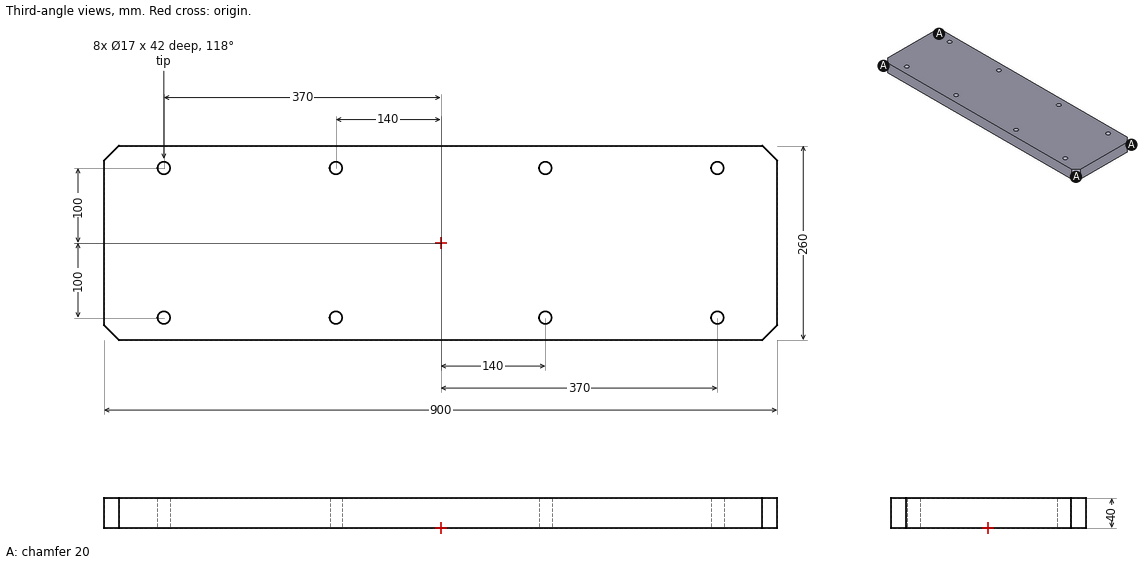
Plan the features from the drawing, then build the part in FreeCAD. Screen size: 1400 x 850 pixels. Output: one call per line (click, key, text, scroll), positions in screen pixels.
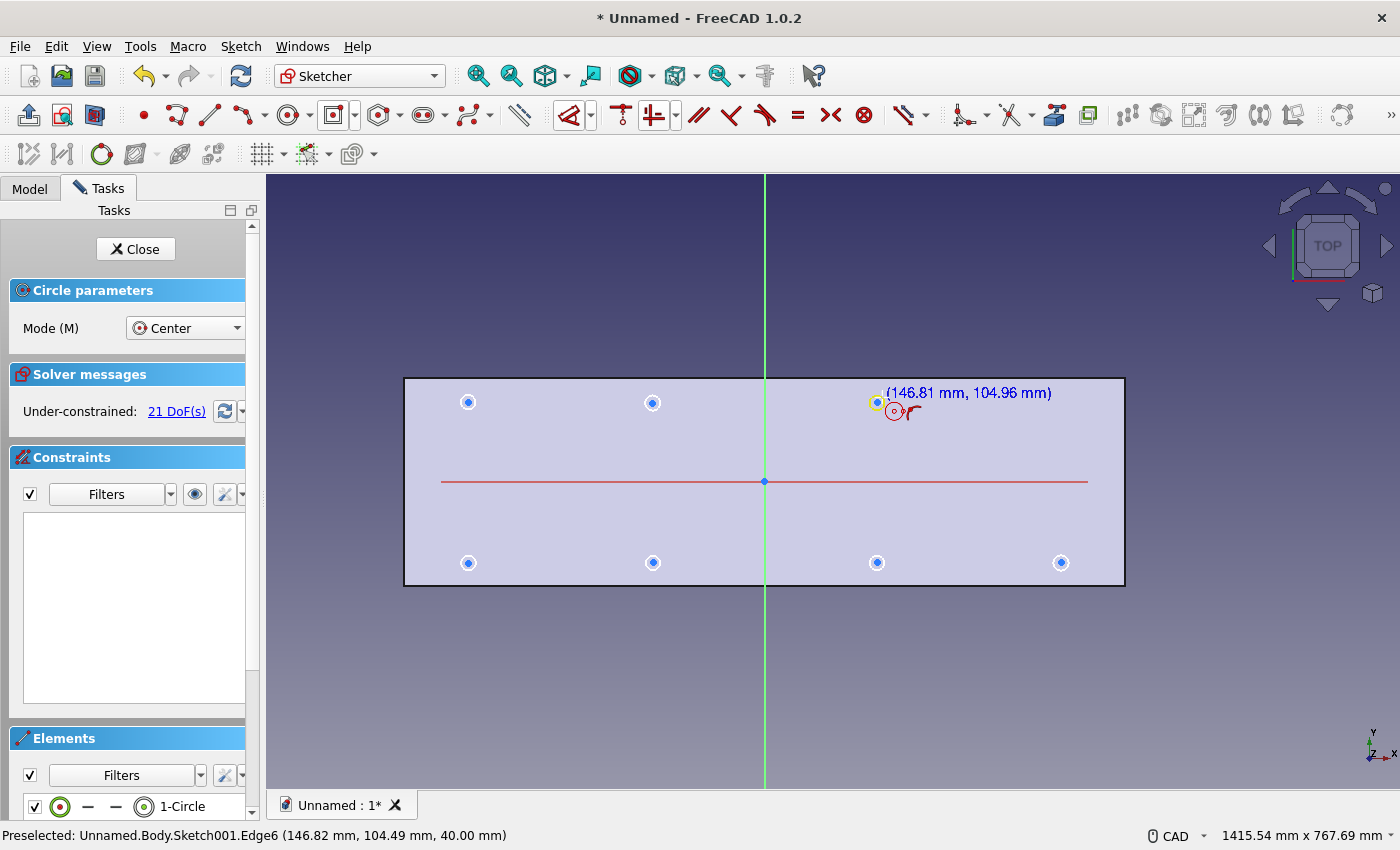
scroll(1061, 402, up, 7)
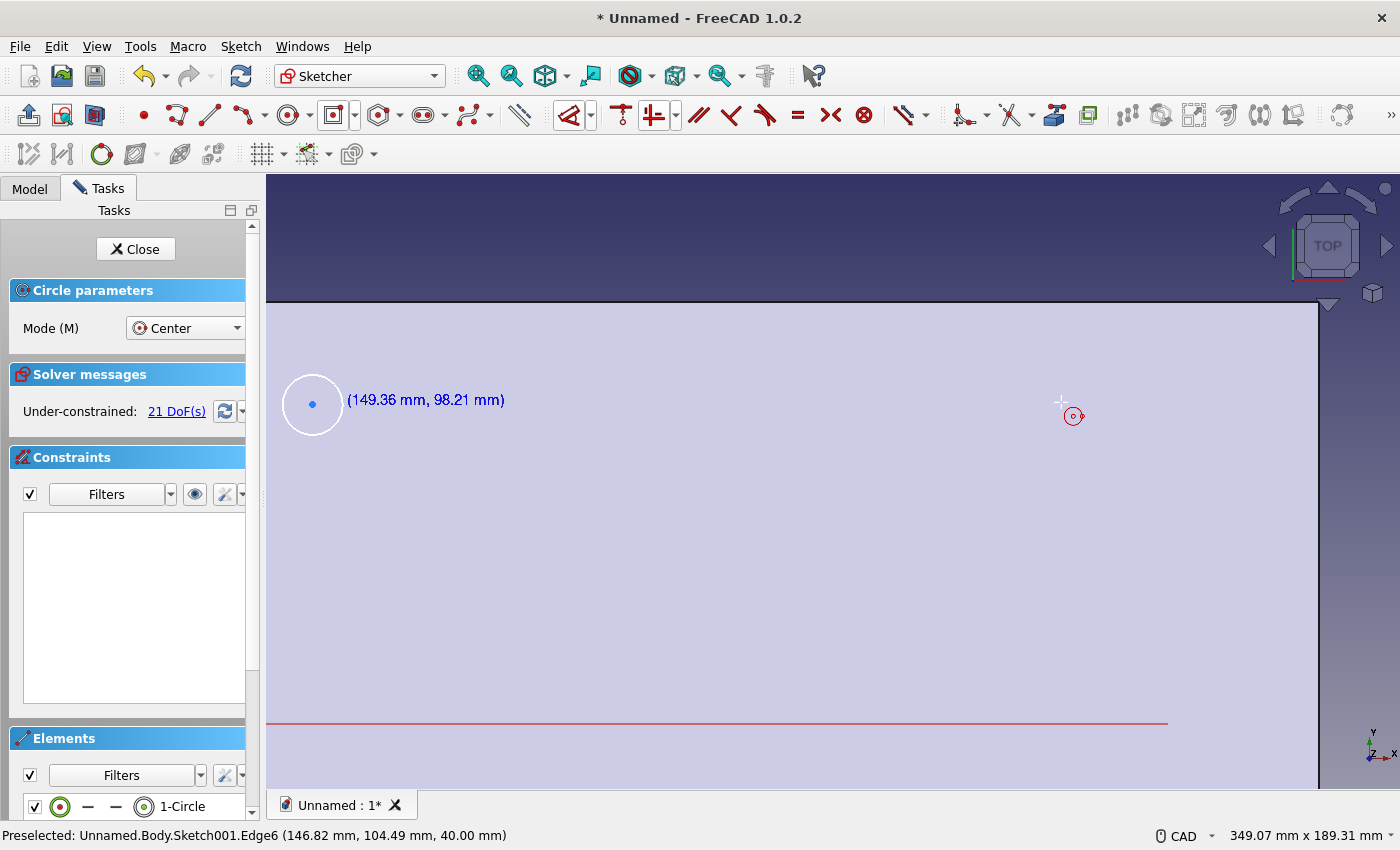
scroll(1061, 402, down, 7)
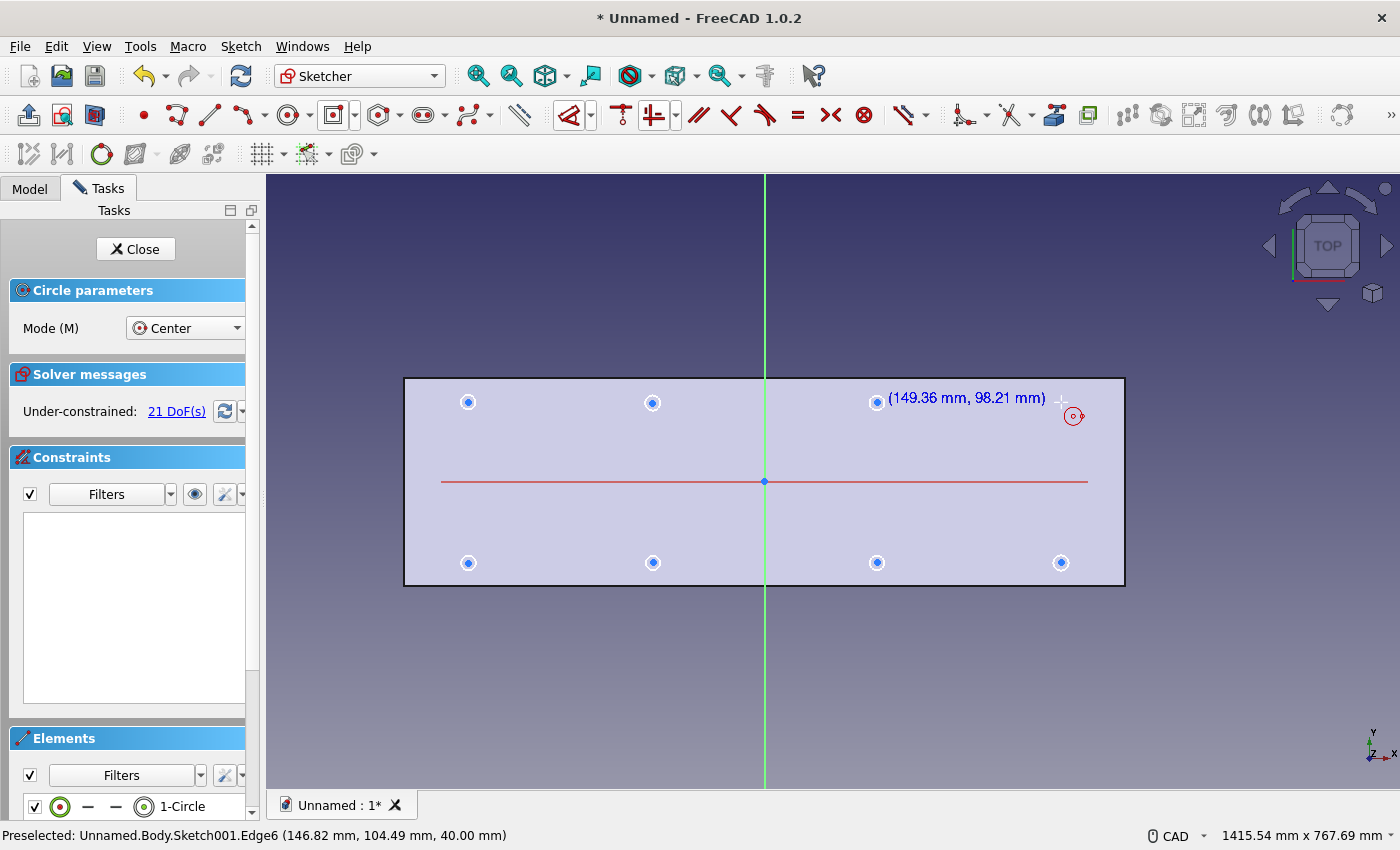
click(1061, 402)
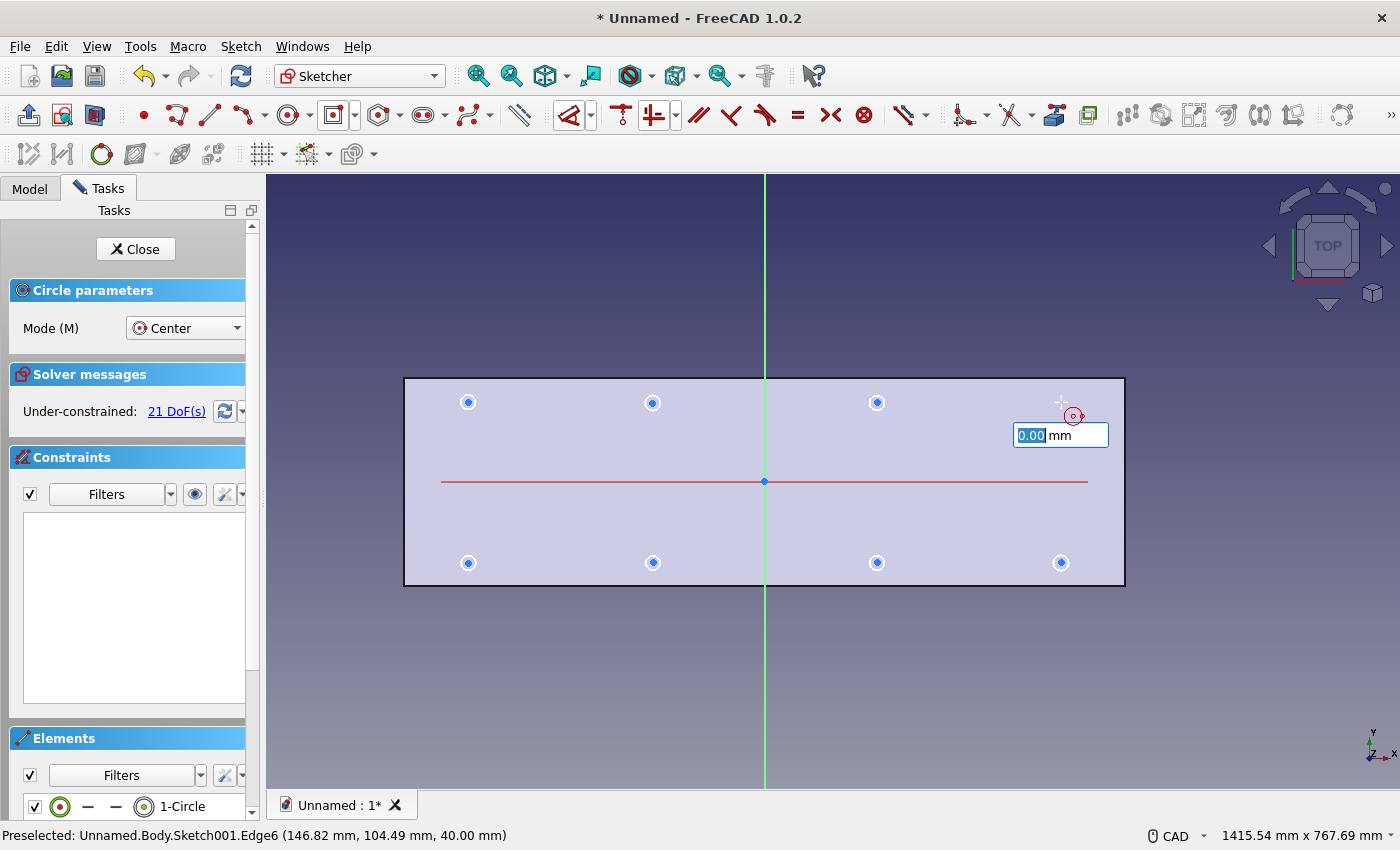
scroll(1066, 397, up, 5)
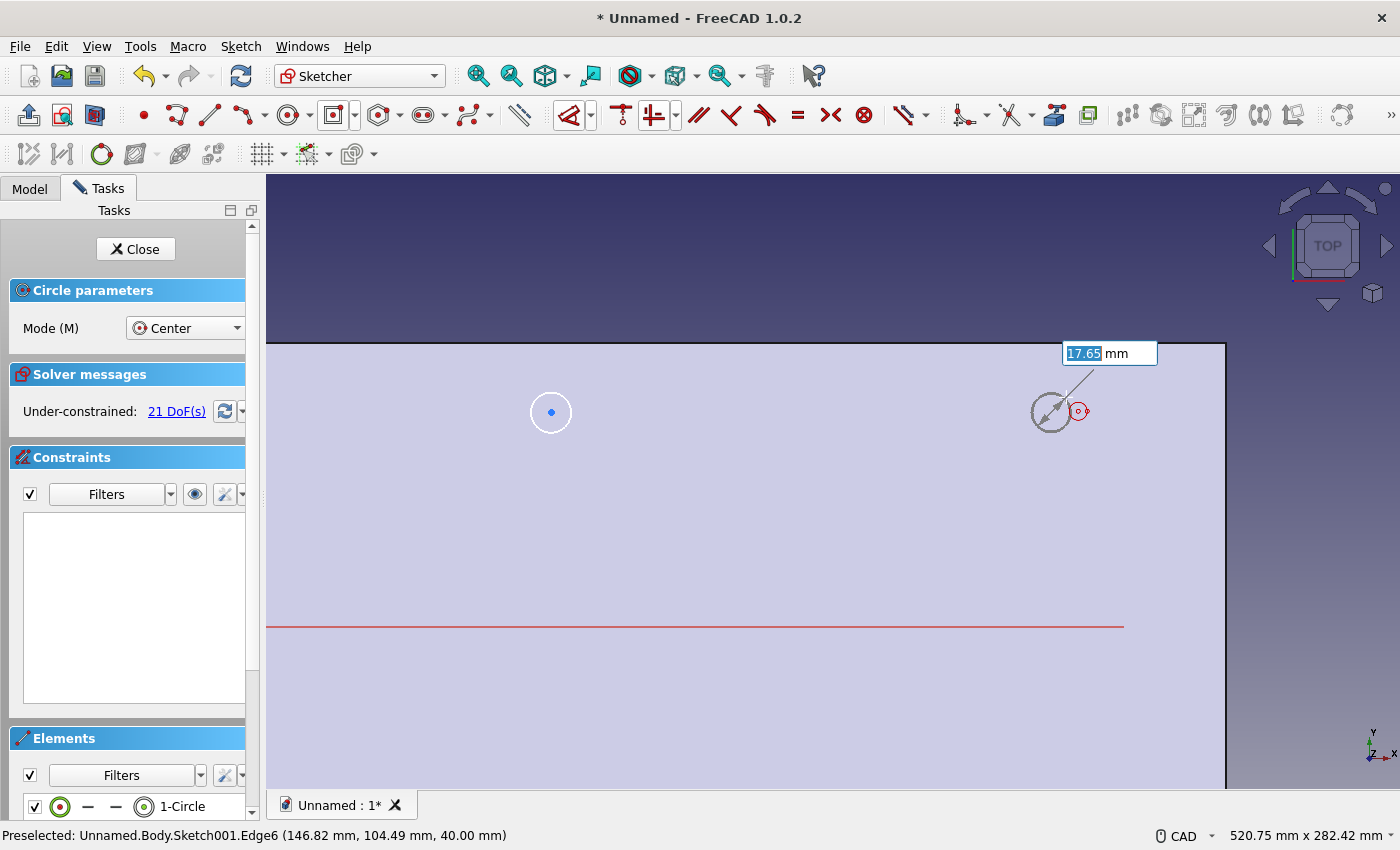
click(1065, 396)
key(Escape)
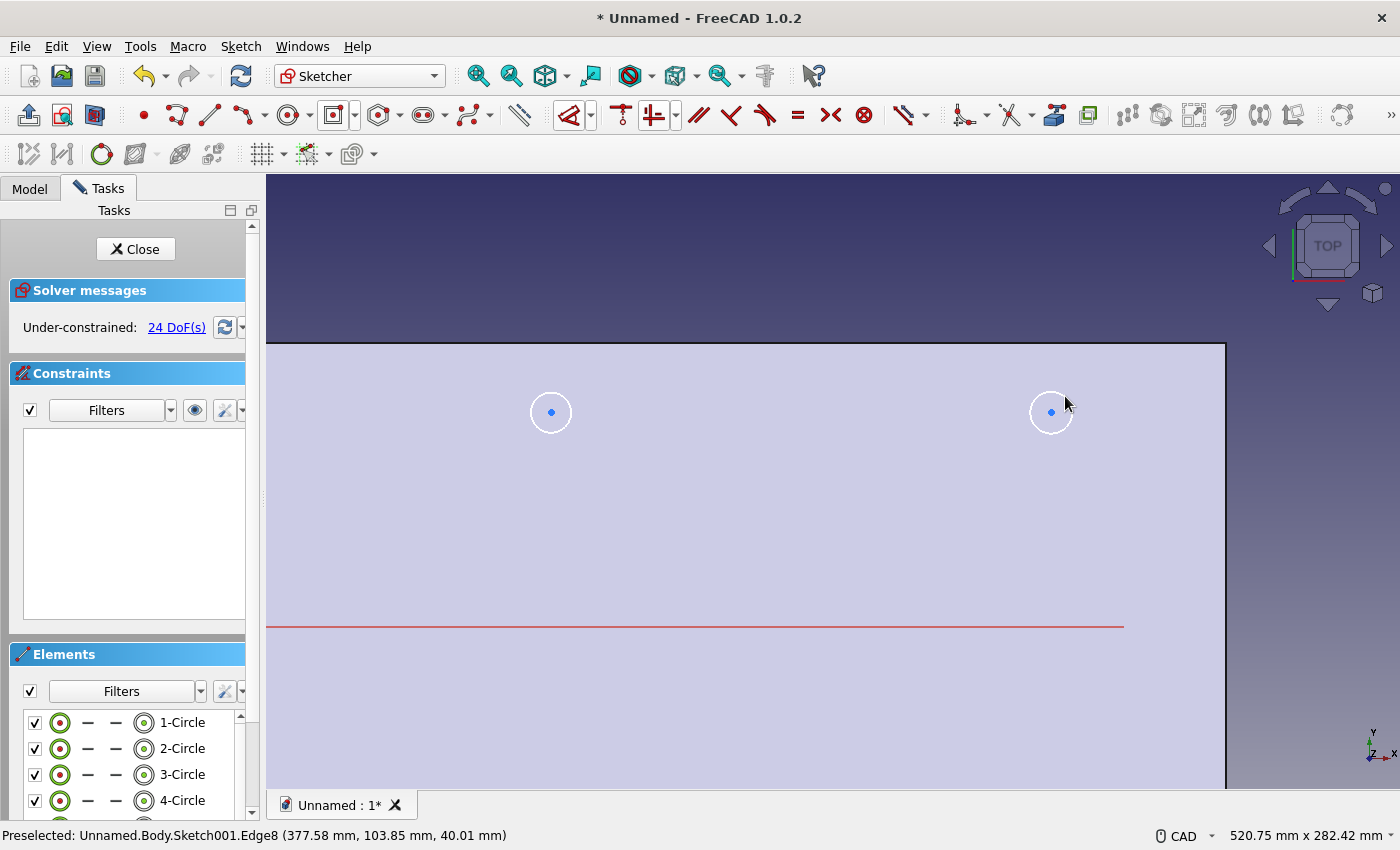
scroll(1066, 397, down, 5)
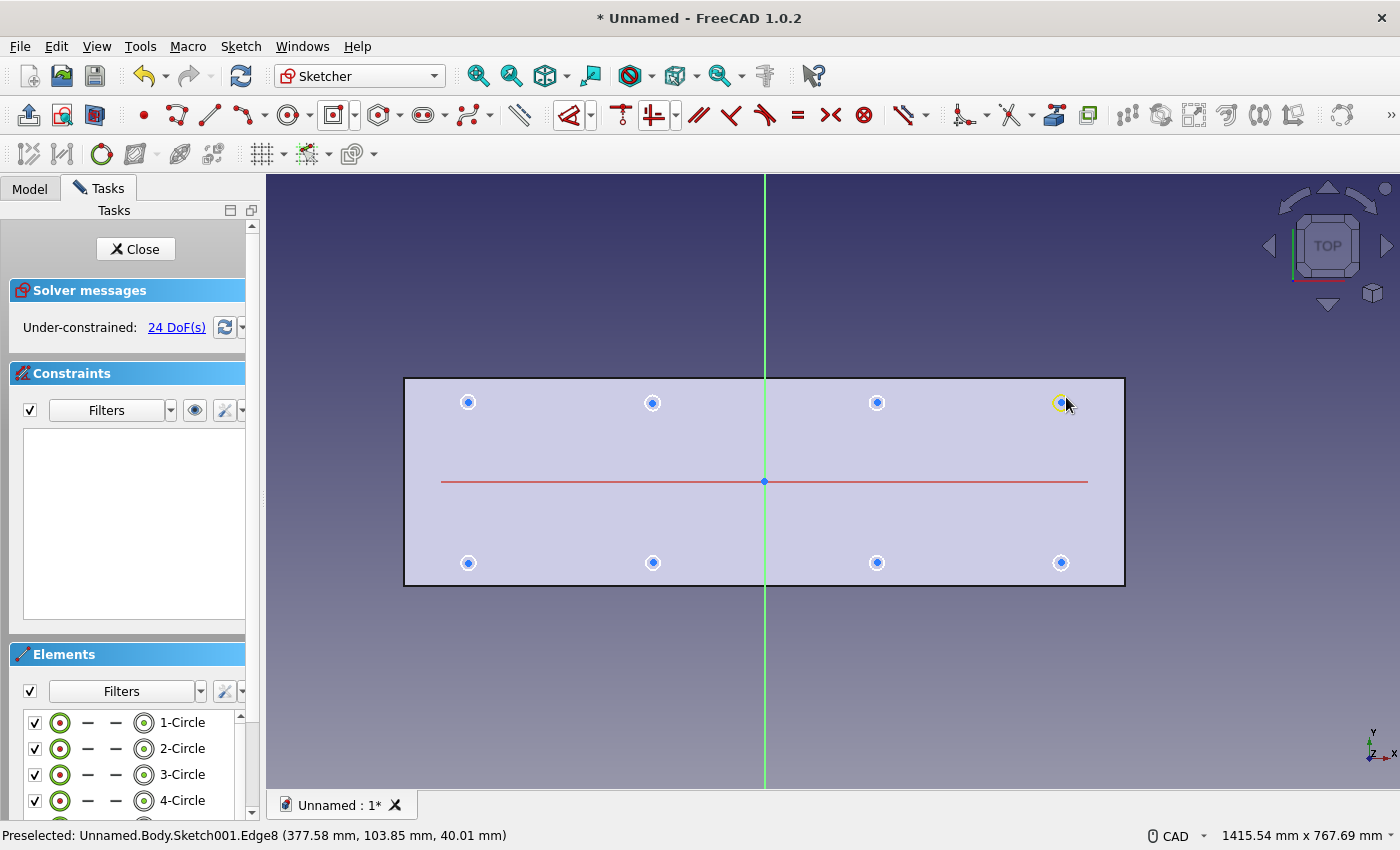
scroll(473, 397, up, 4)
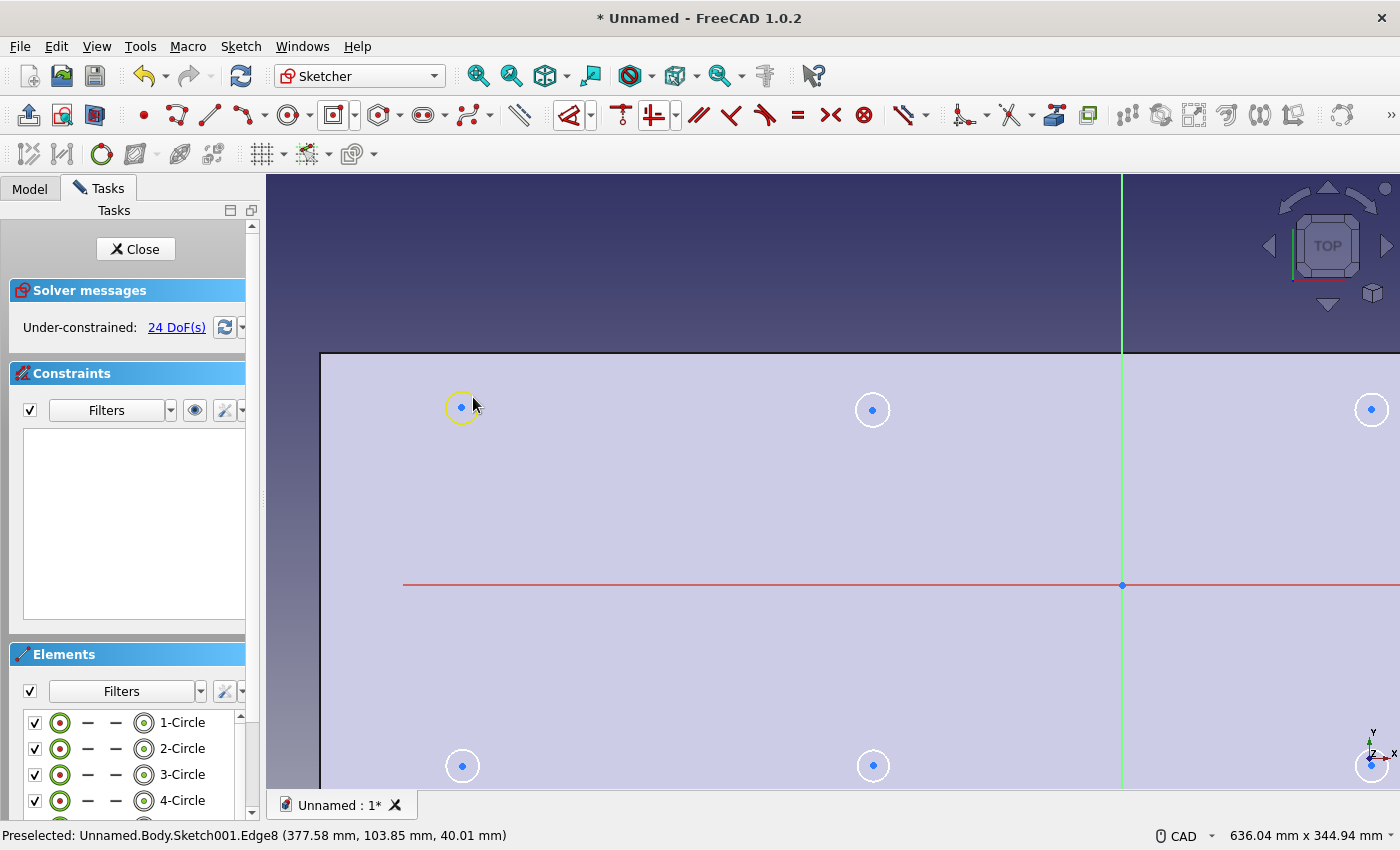
click(473, 396)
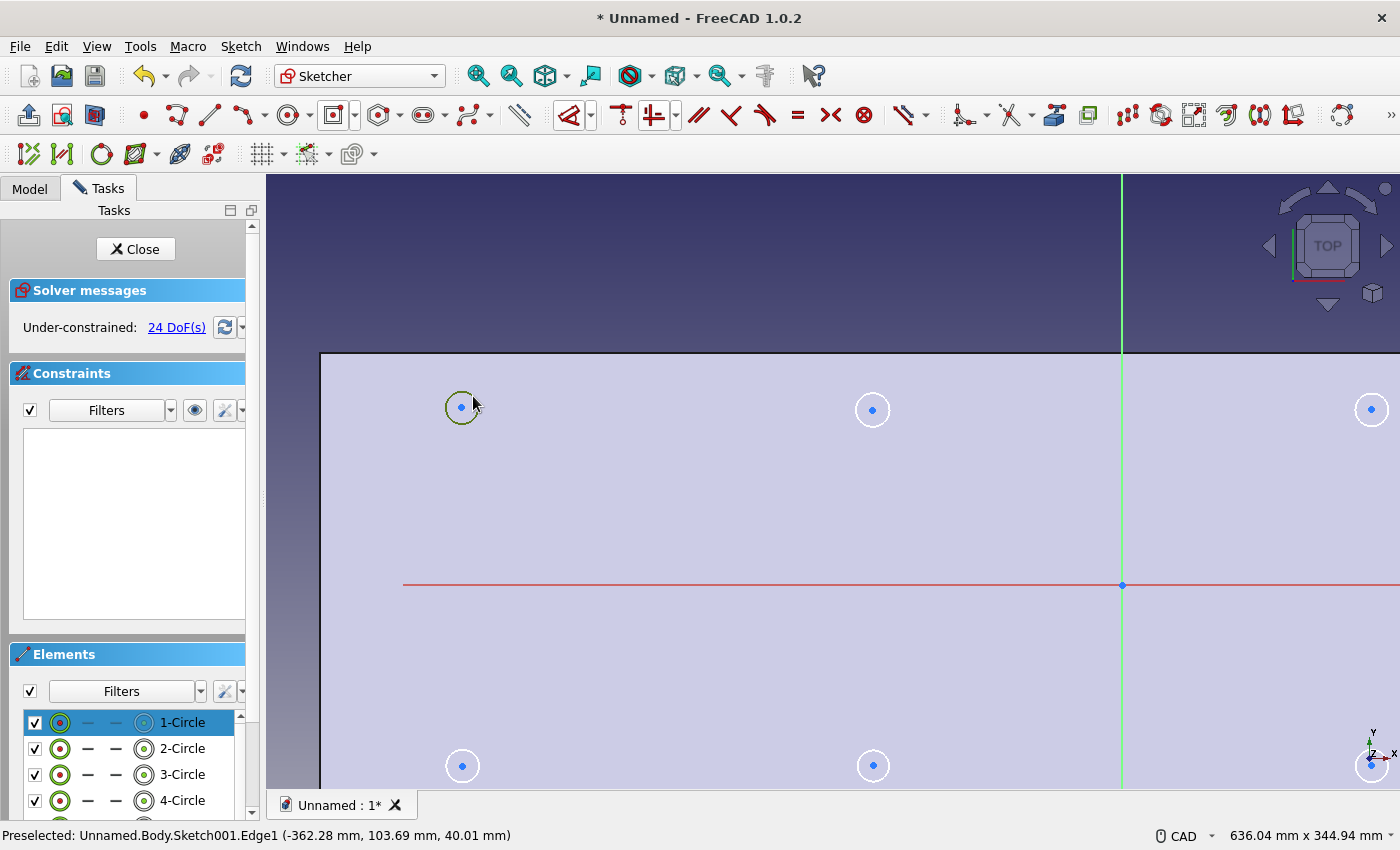
click(885, 398)